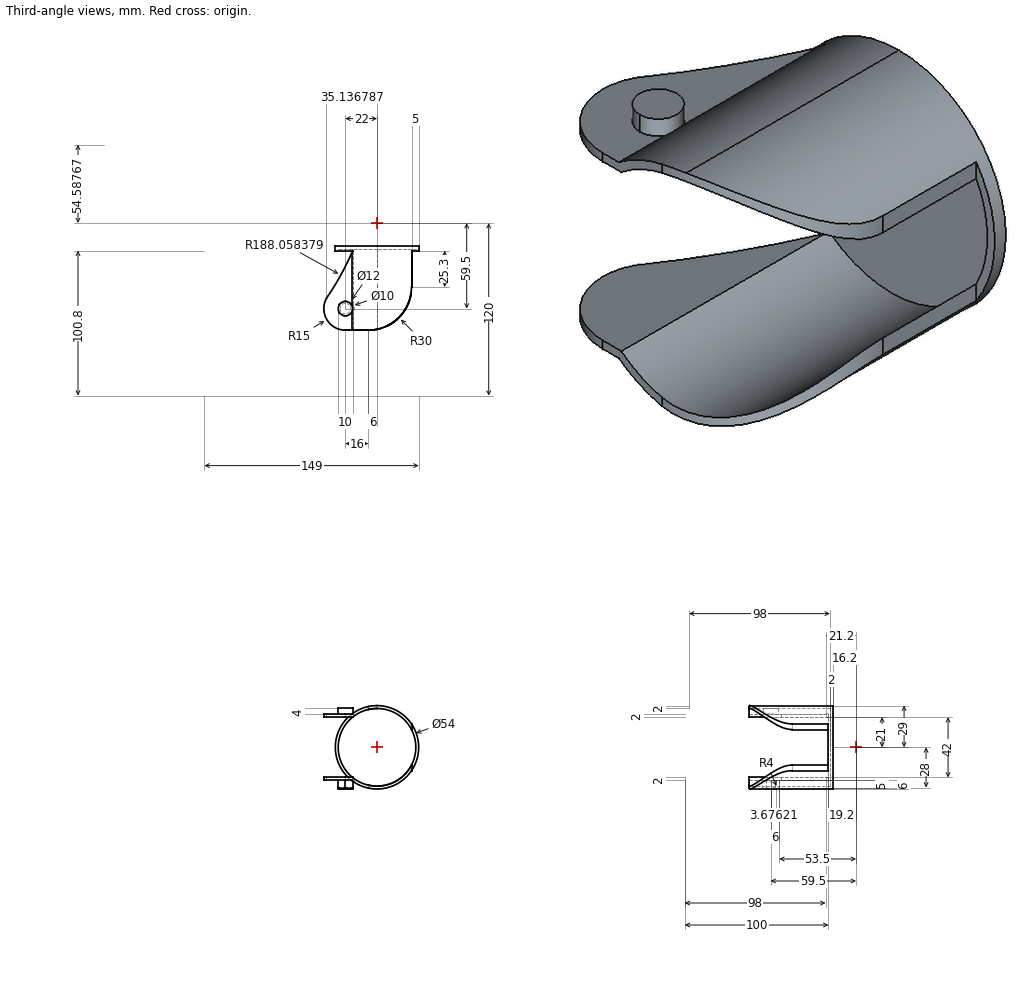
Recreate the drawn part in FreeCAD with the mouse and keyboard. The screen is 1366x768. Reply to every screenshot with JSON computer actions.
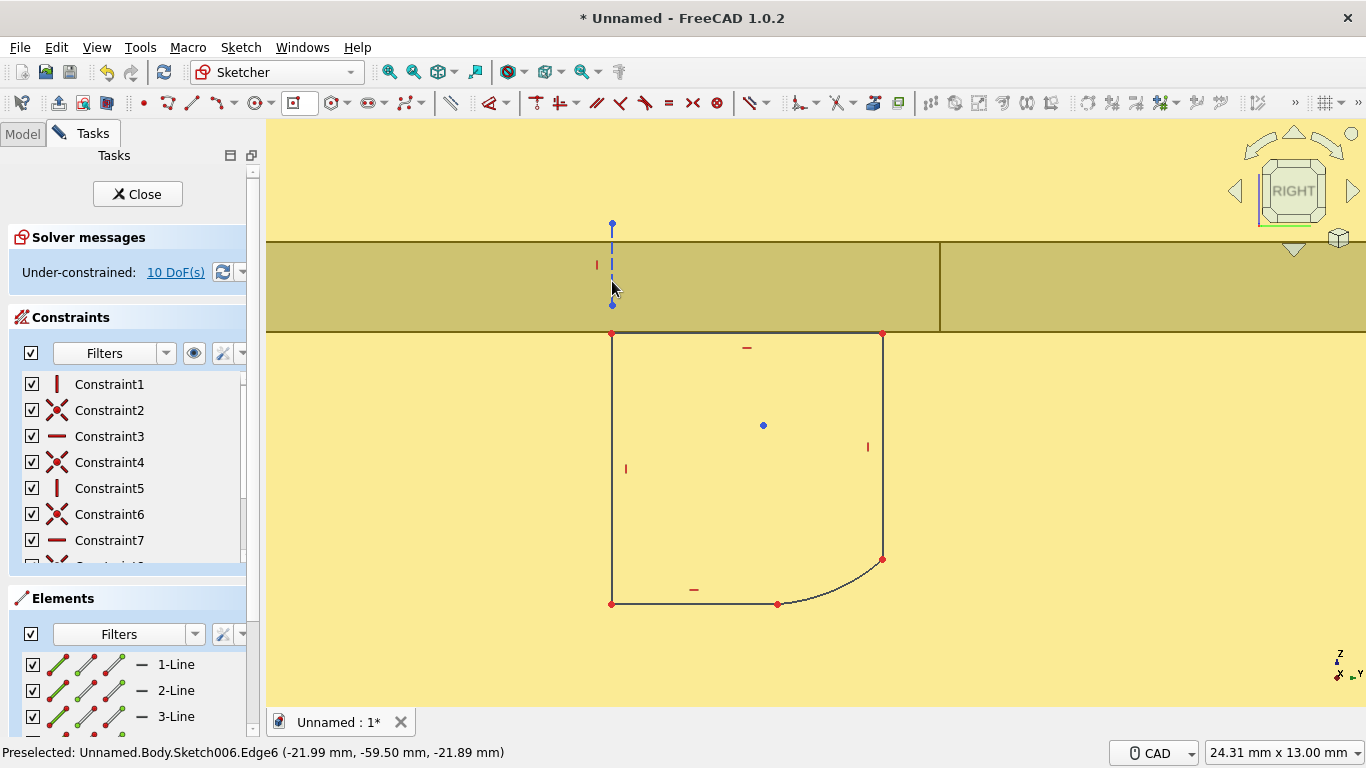
{"action": "key", "text": "d"}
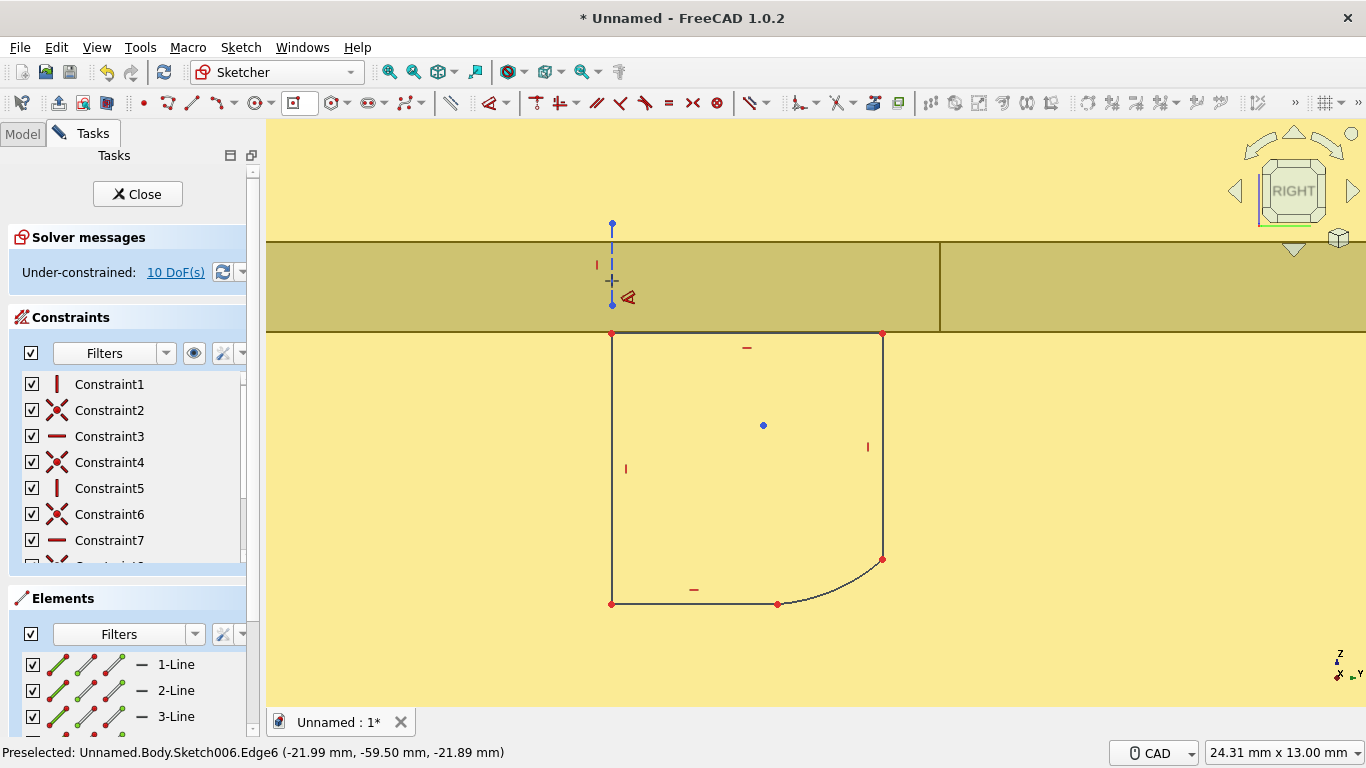
{"action": "left_click", "coordinate": [812, 598]}
{"action": "left_click", "coordinate": [821, 629]}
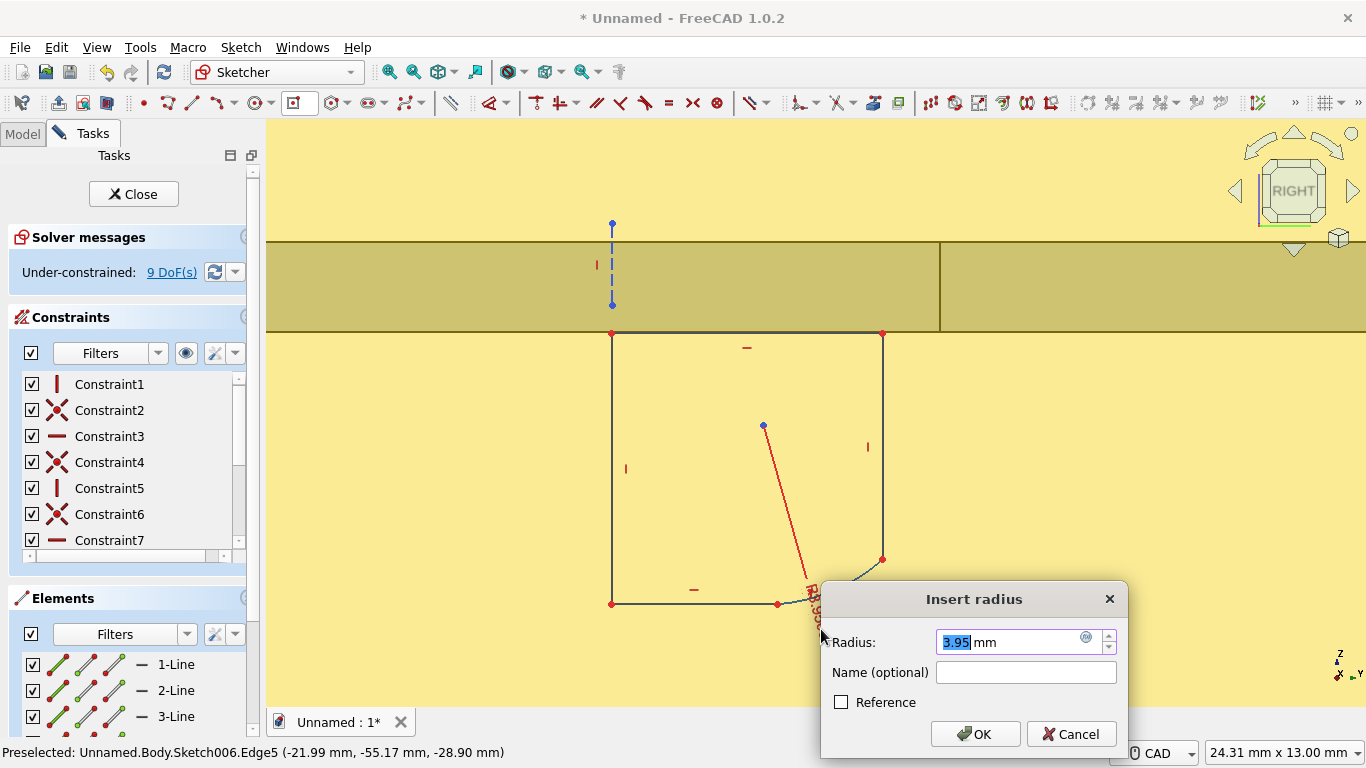
{"action": "type", "text": "4"}
{"action": "key", "text": "Return"}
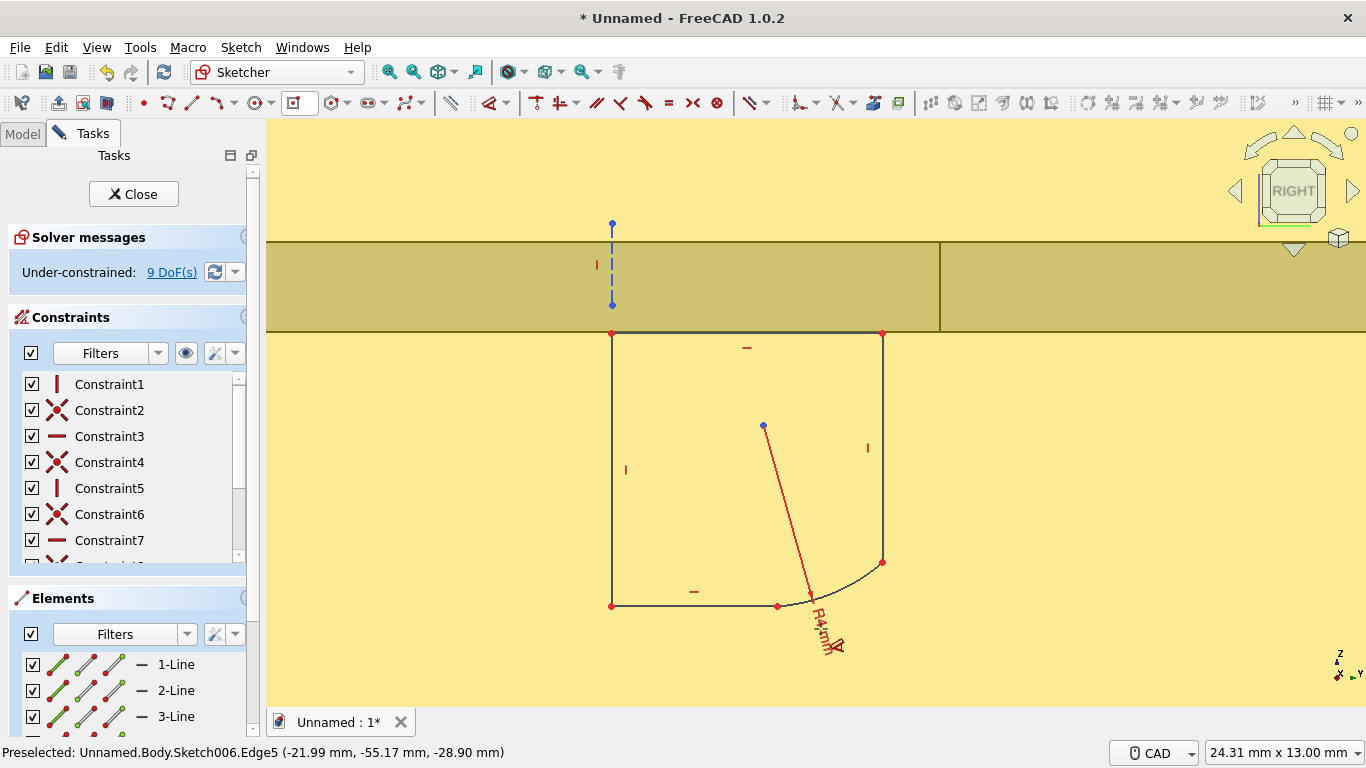
{"action": "left_click", "coordinate": [883, 493]}
{"action": "left_click", "coordinate": [917, 448]}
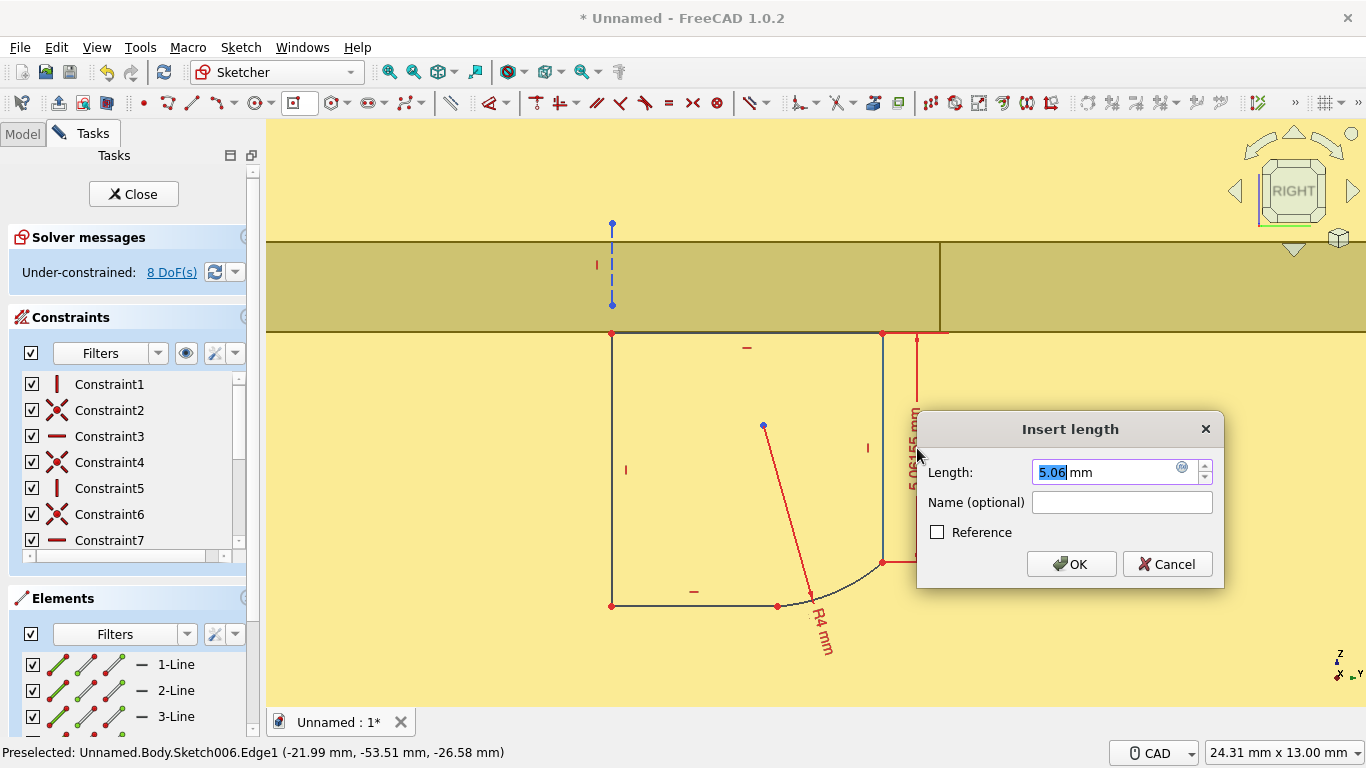
{"action": "type", "text": "5"}
{"action": "key", "text": "Return"}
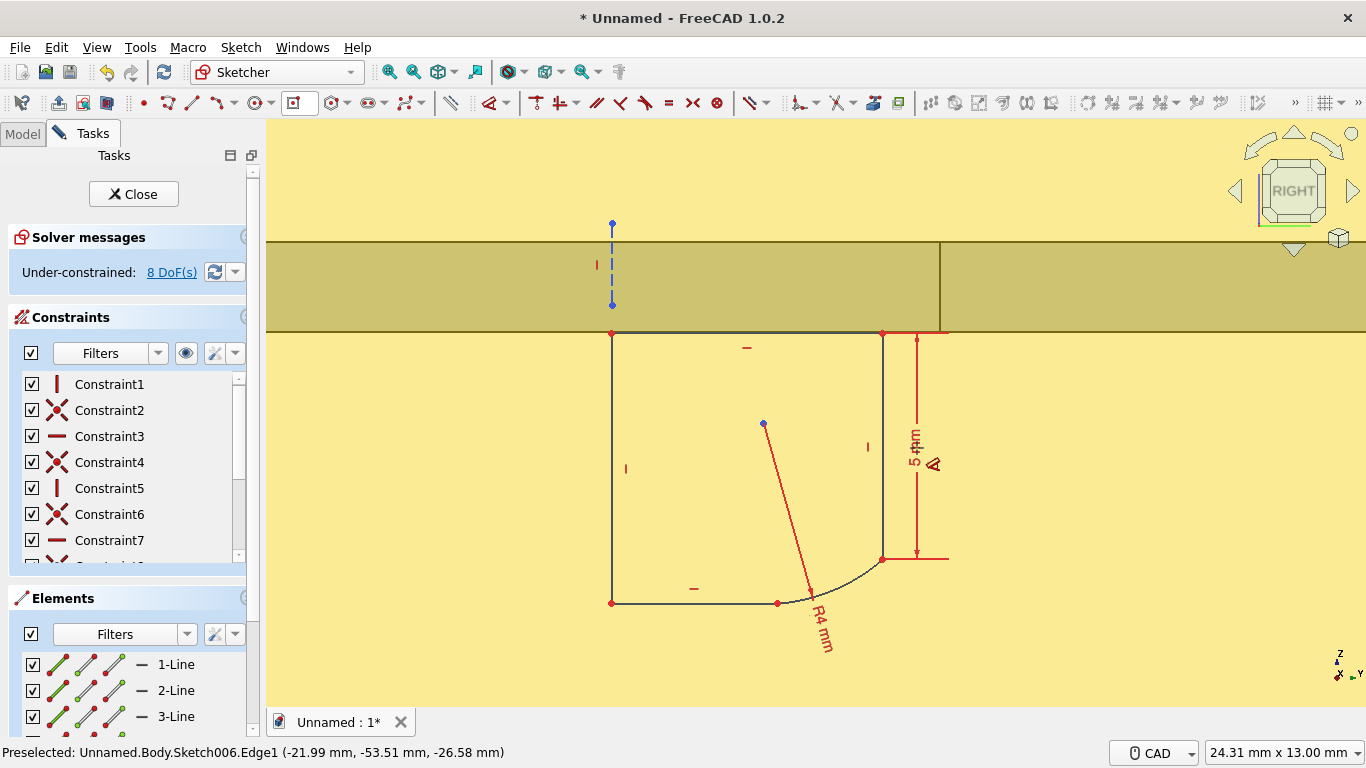
{"action": "left_click", "coordinate": [802, 333]}
{"action": "left_click", "coordinate": [747, 299]}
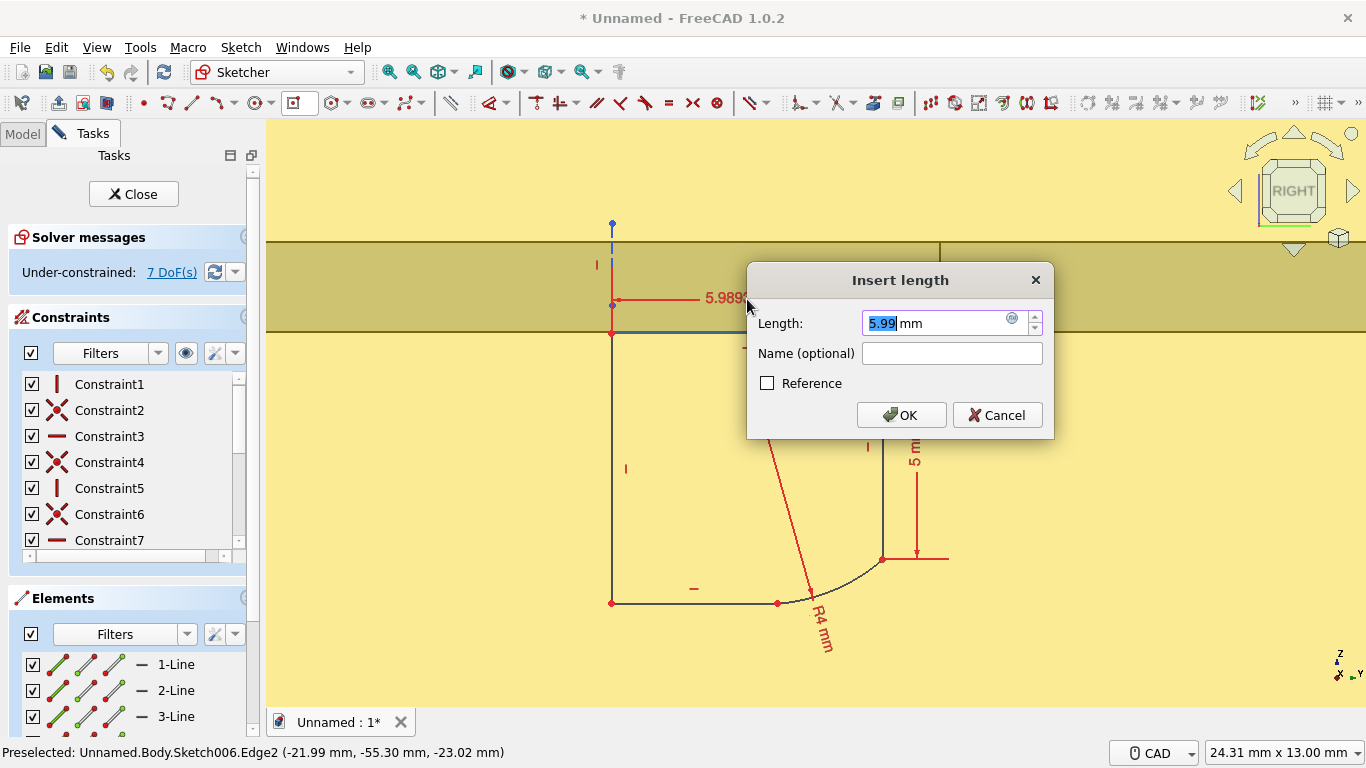
{"action": "type", "text": "6"}
{"action": "key", "text": "Return"}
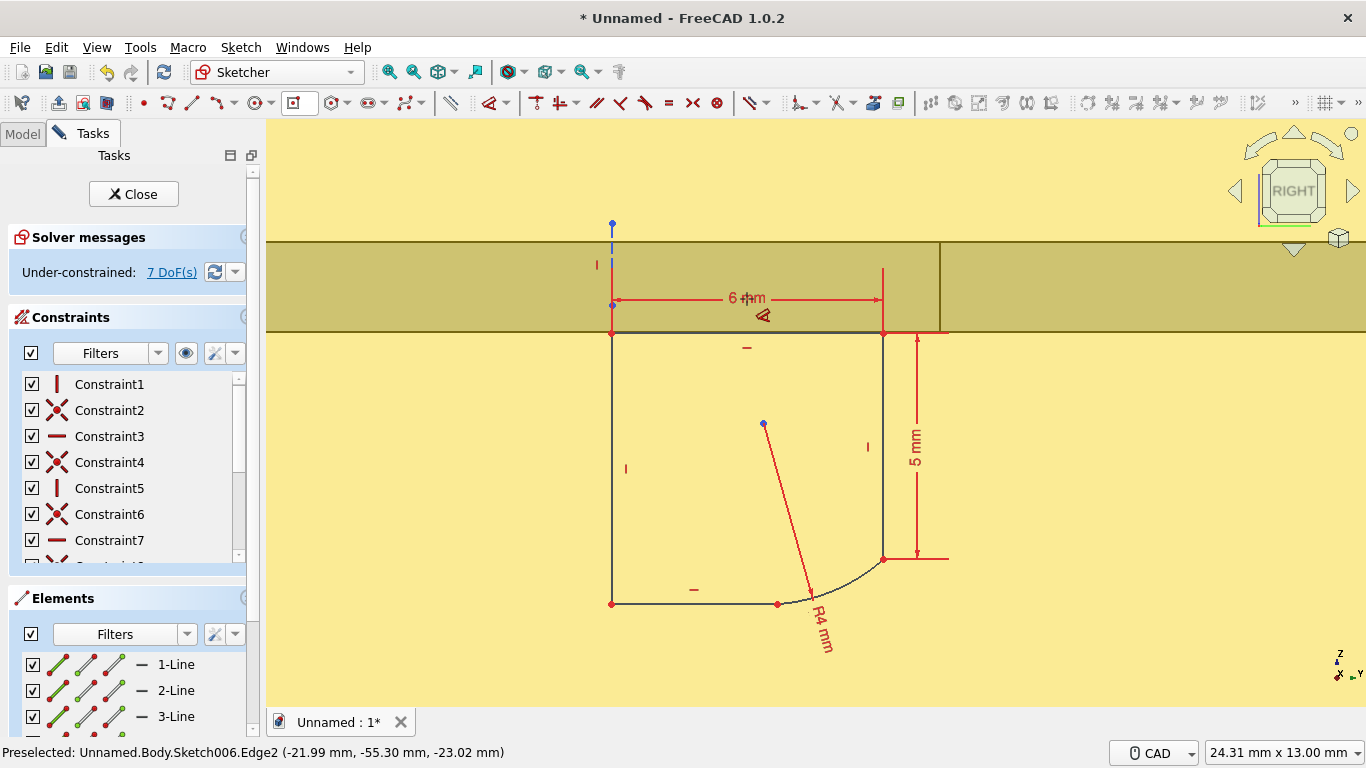
{"action": "left_click", "coordinate": [612, 414]}
{"action": "left_click", "coordinate": [578, 469]}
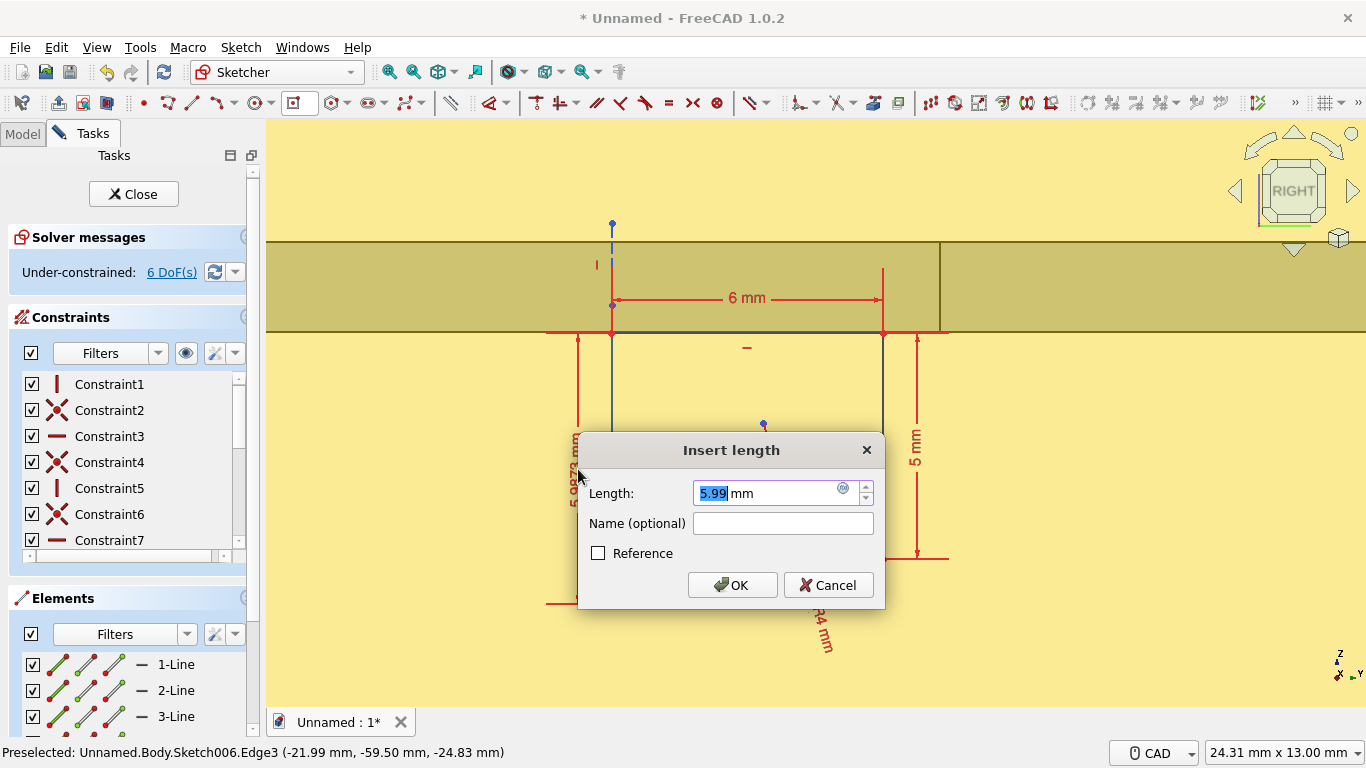
{"action": "type", "text": "6"}
{"action": "key", "text": "Return"}